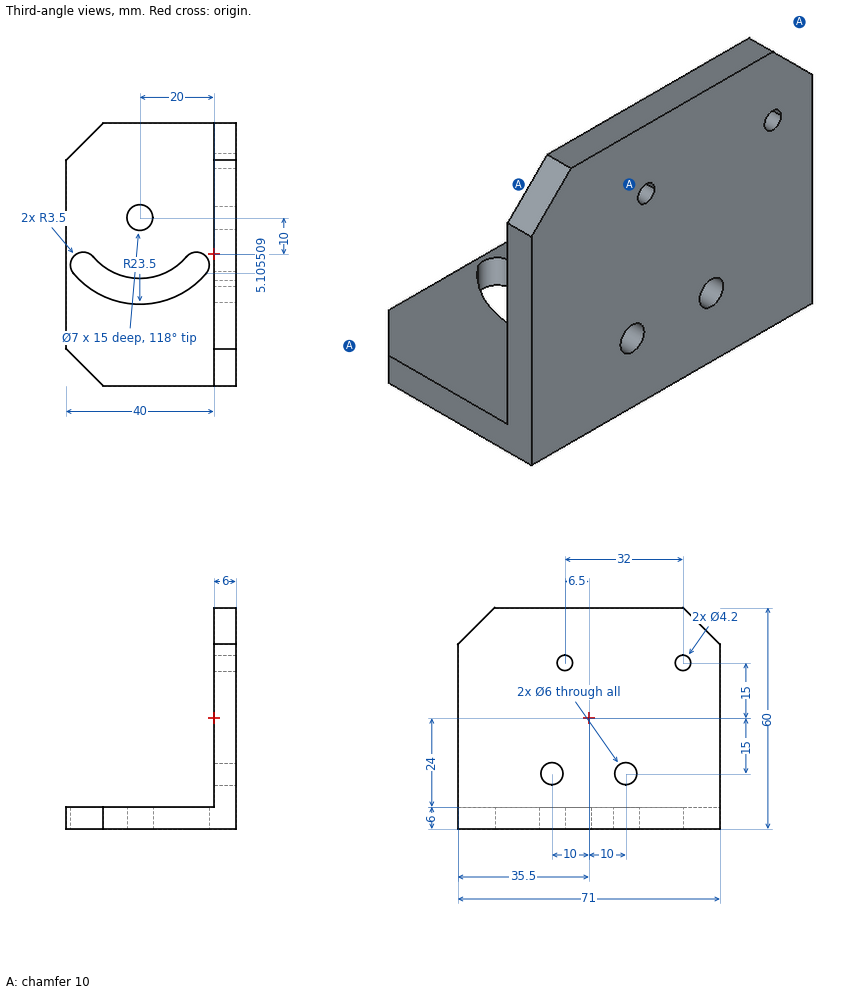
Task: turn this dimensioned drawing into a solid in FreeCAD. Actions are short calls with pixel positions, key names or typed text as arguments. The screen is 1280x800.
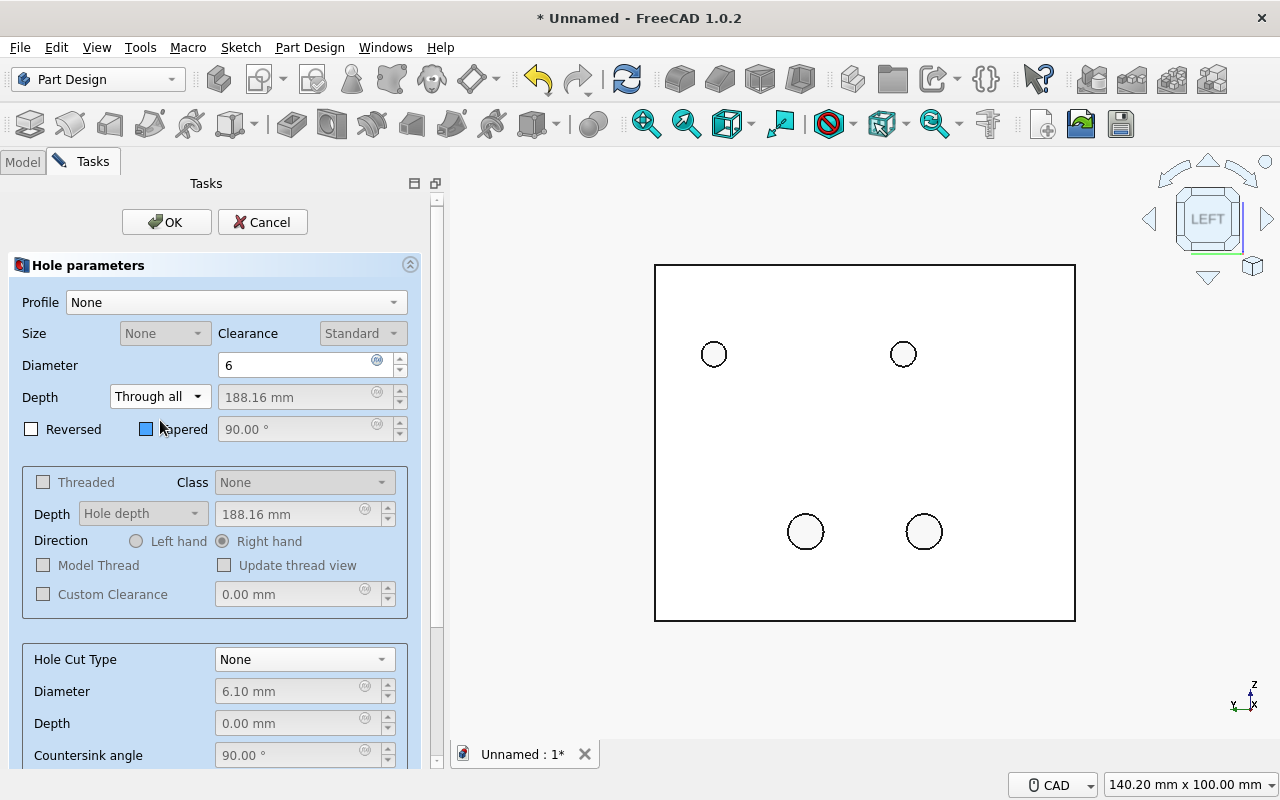
click(167, 222)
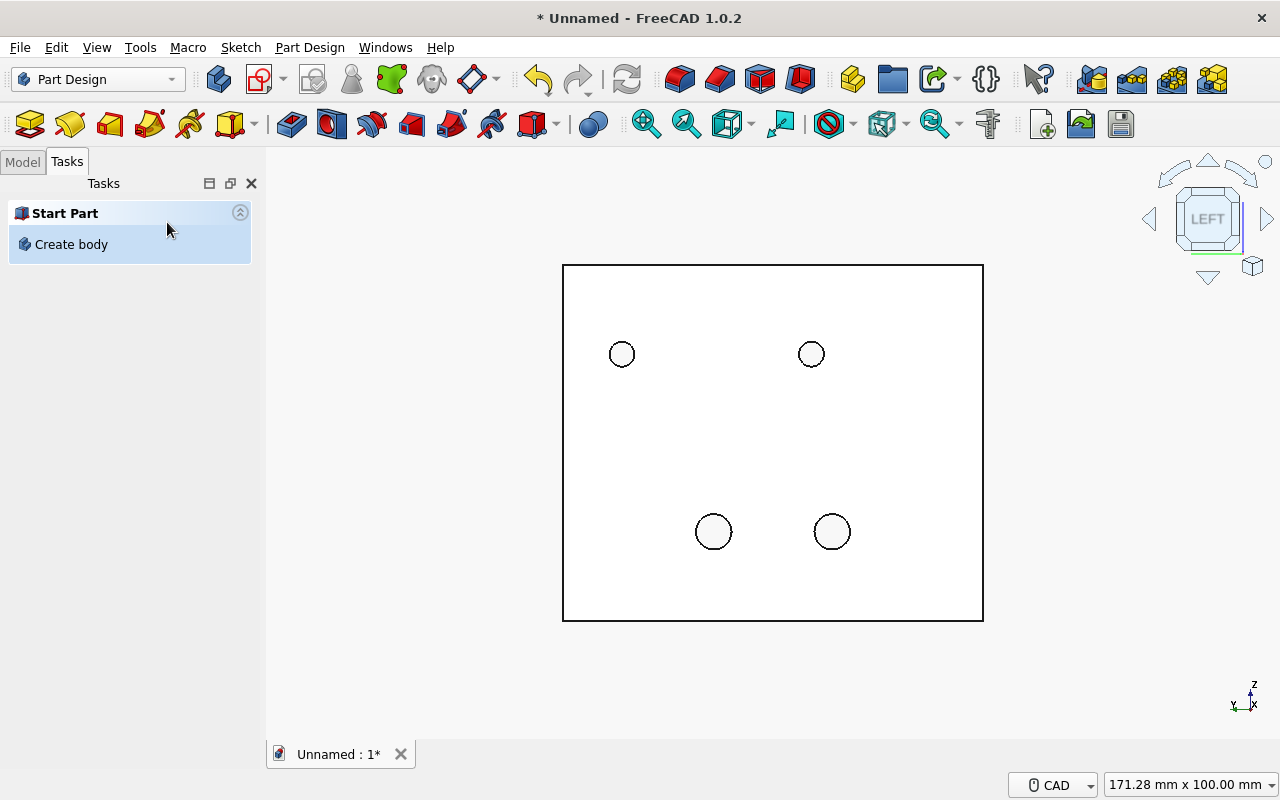
click(260, 80)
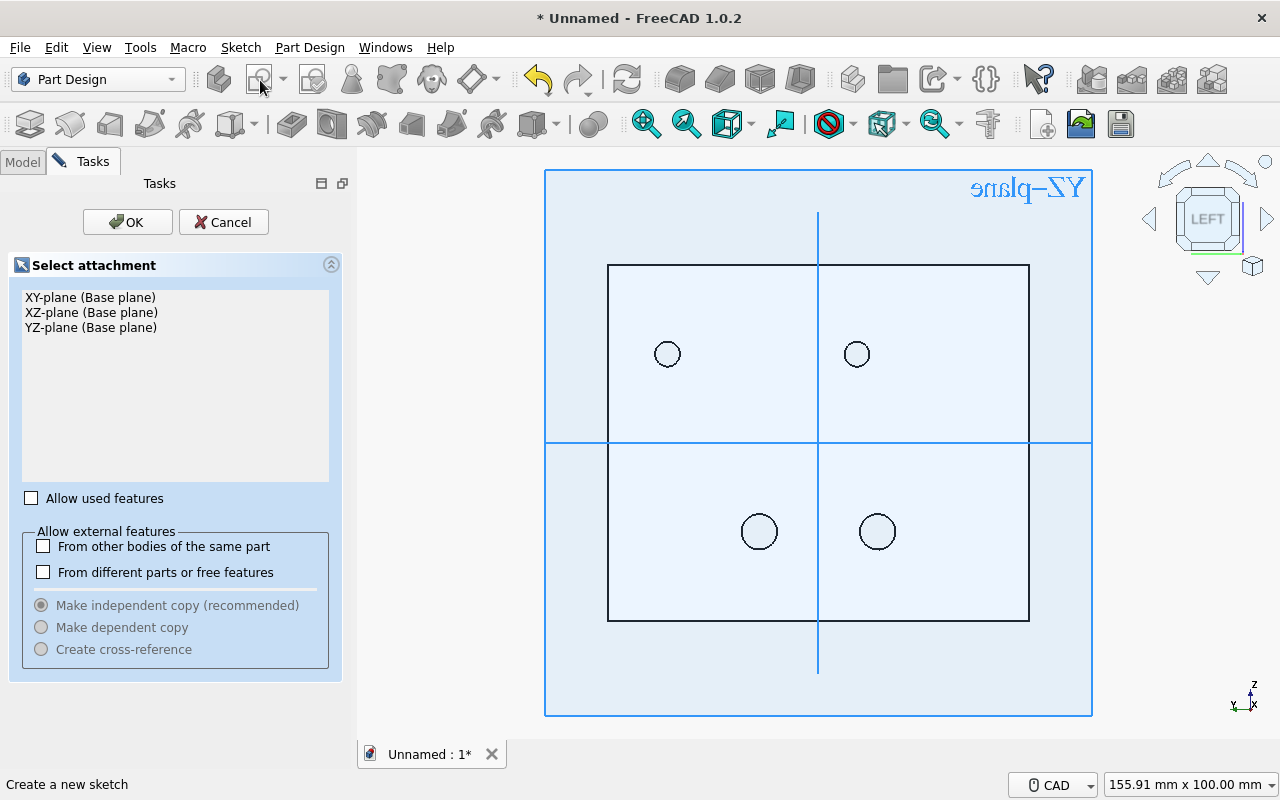
click(82, 328)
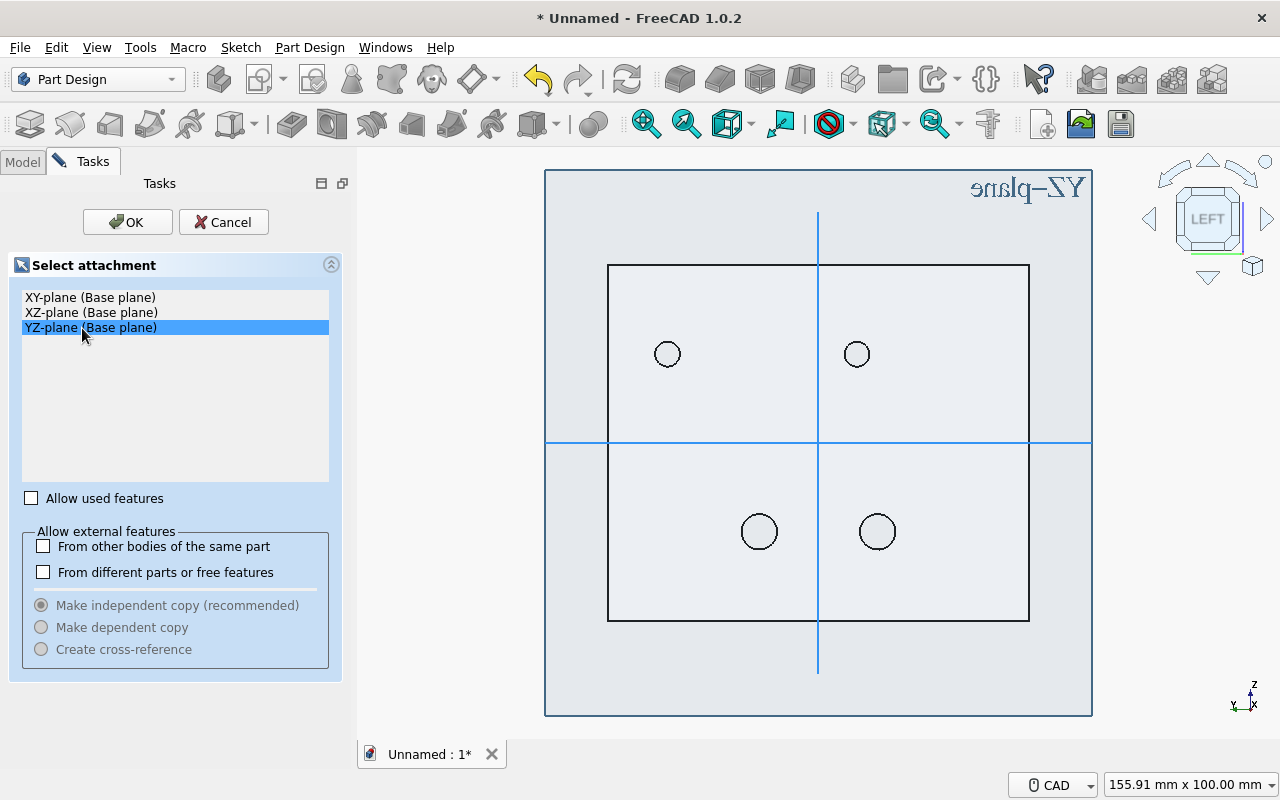
click(128, 222)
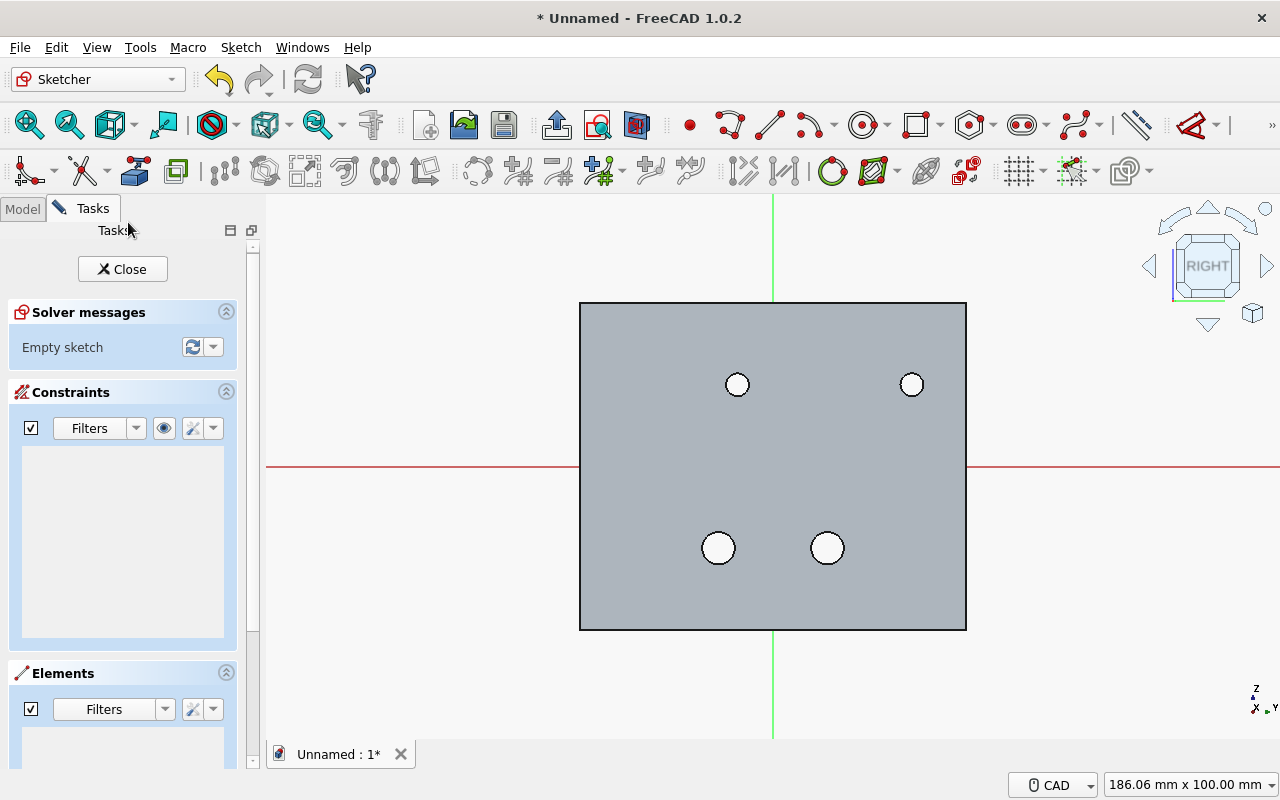
click(638, 126)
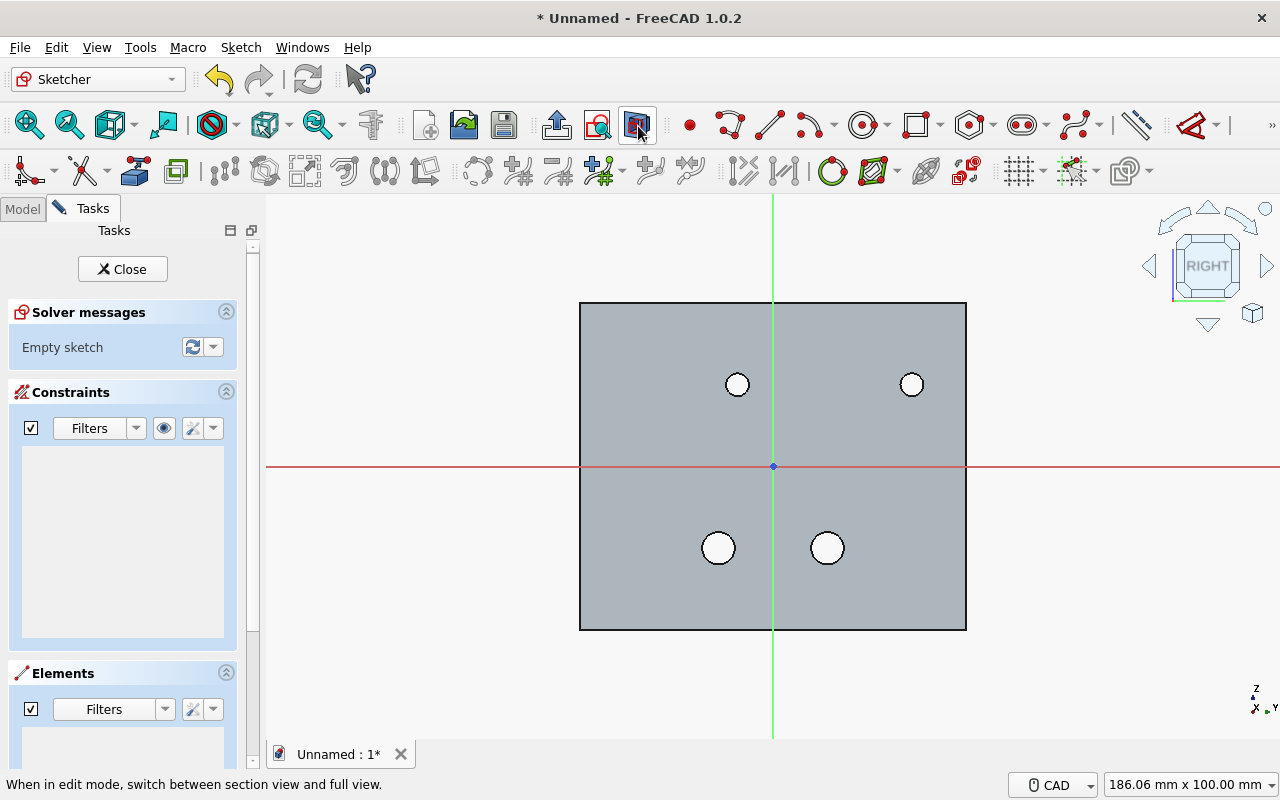
scroll(912, 711, up, 2)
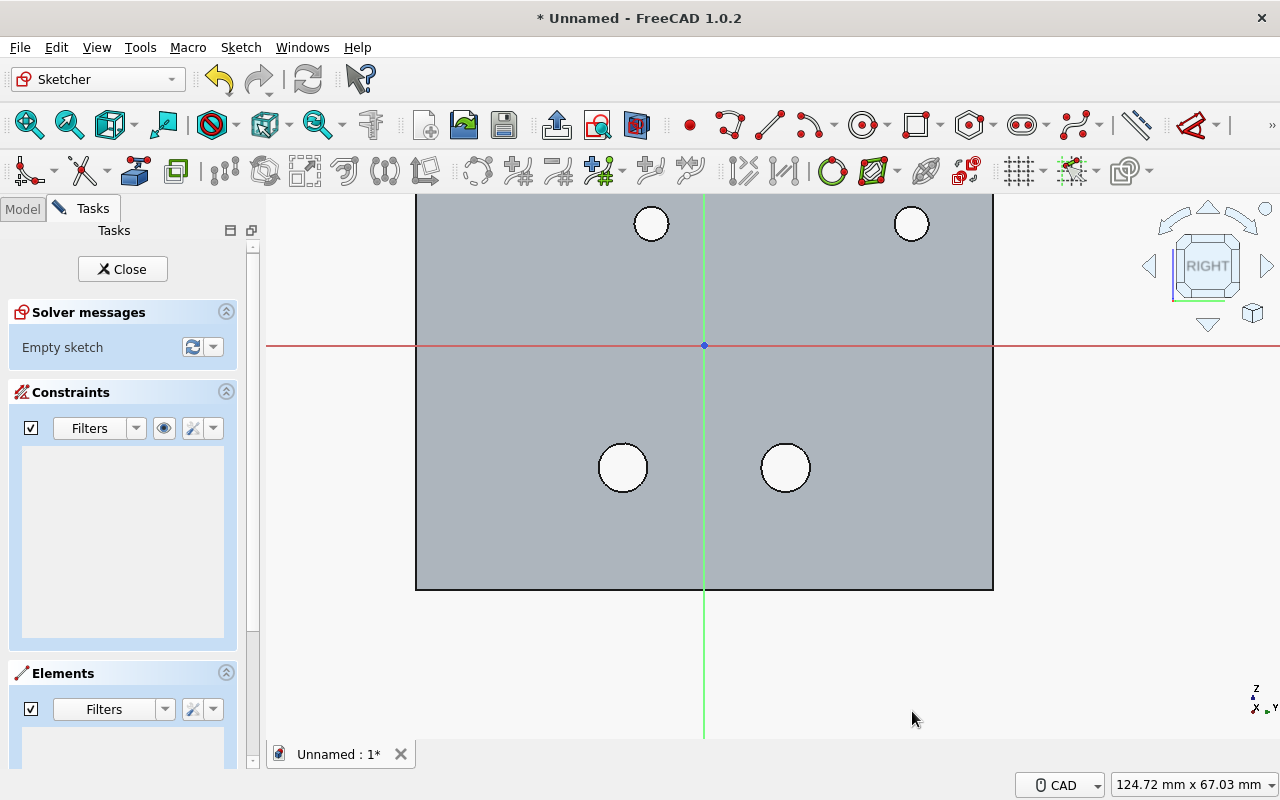
click(916, 126)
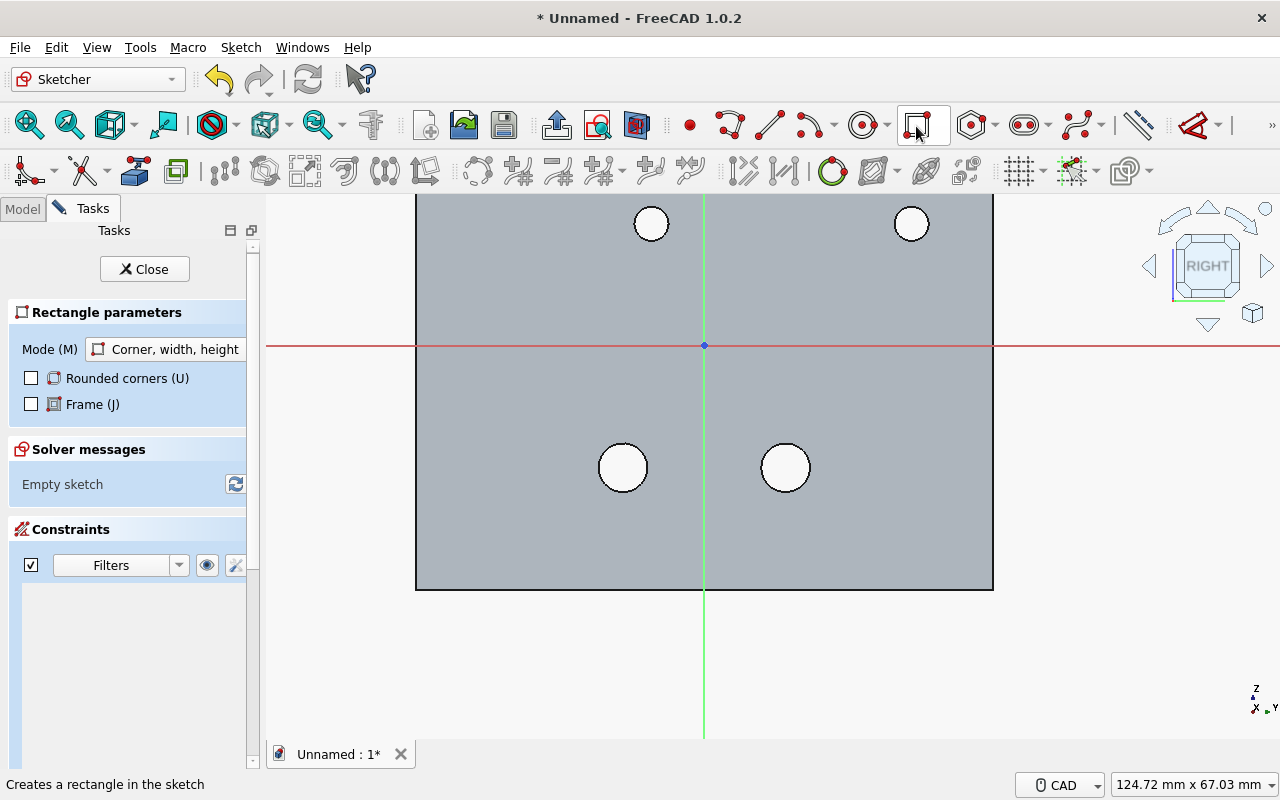
click(416, 541)
click(993, 590)
key(Escape)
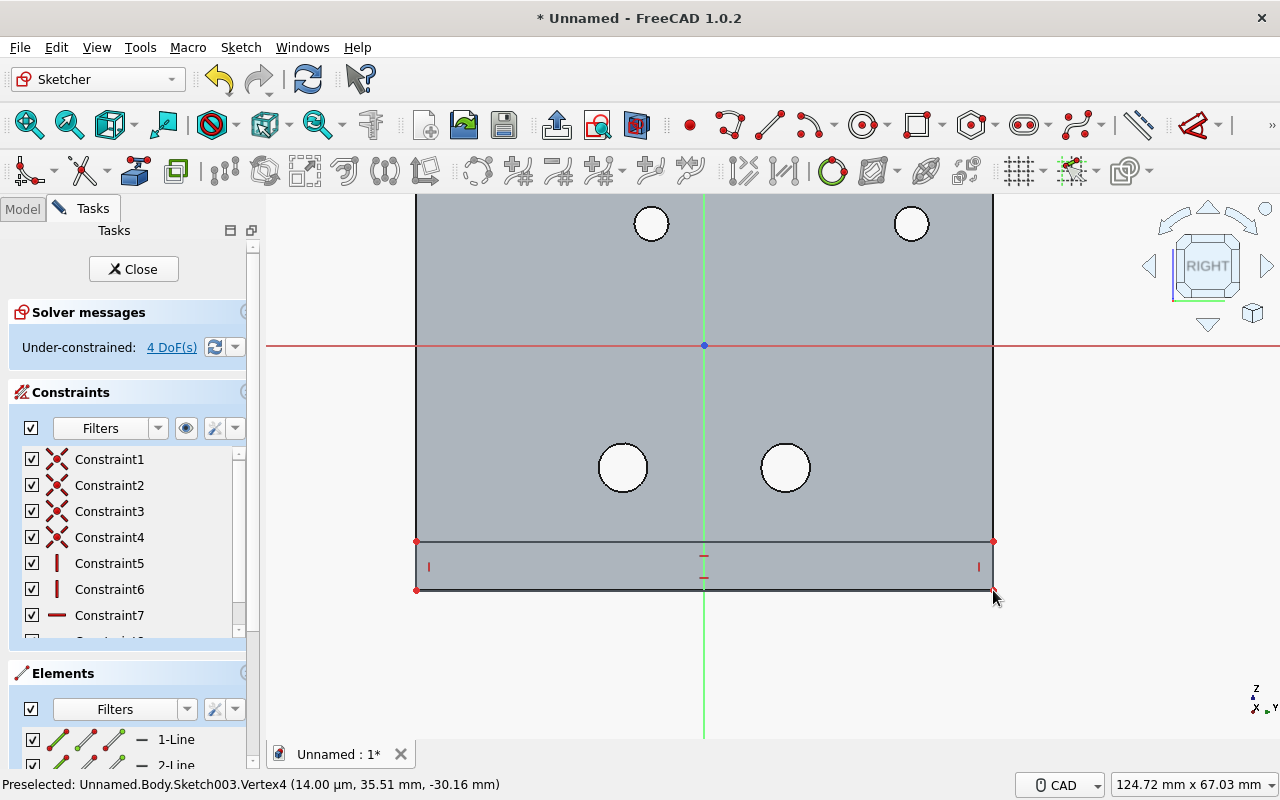
click(1194, 126)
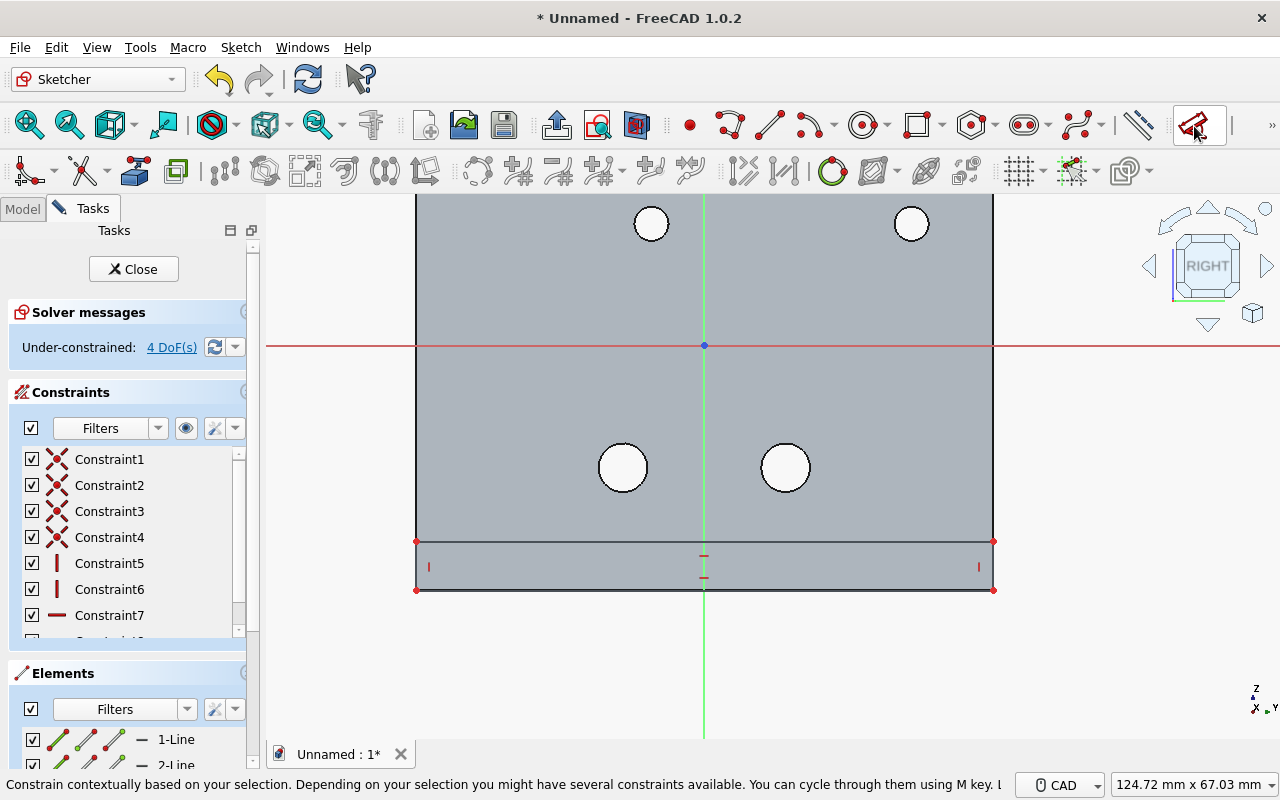
click(416, 557)
click(382, 567)